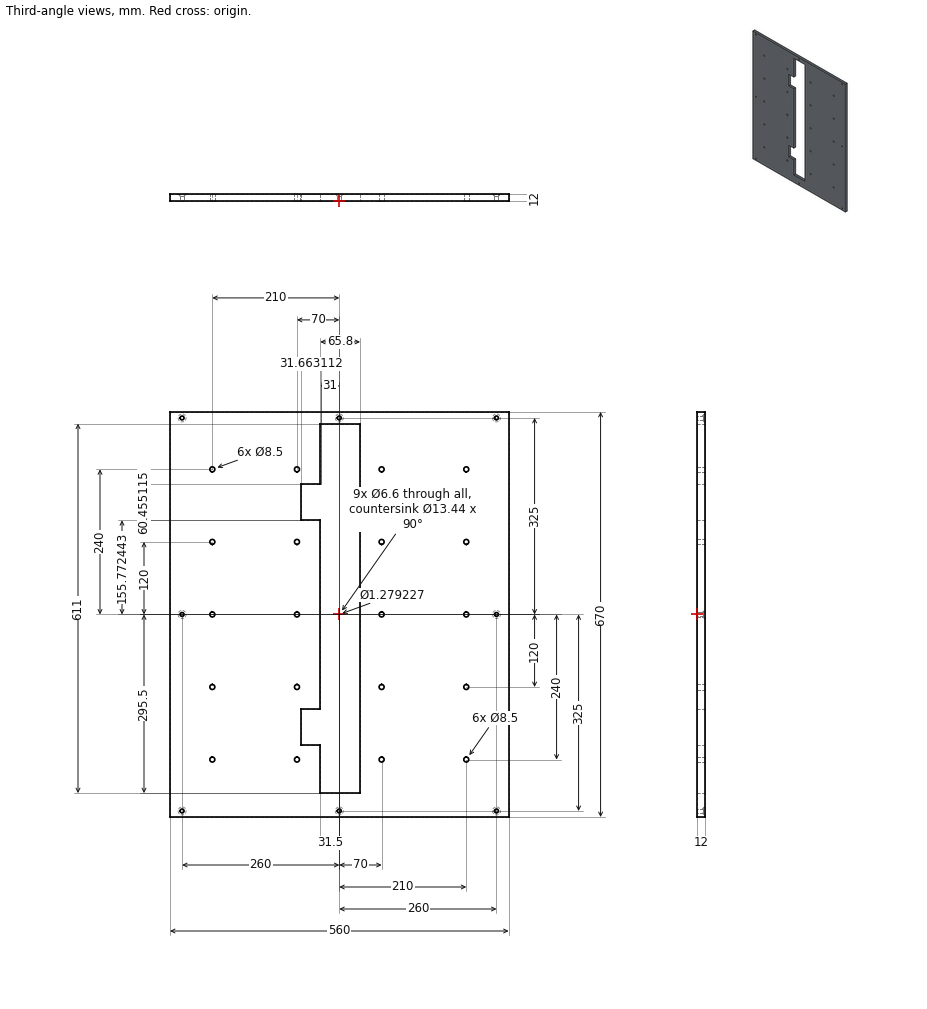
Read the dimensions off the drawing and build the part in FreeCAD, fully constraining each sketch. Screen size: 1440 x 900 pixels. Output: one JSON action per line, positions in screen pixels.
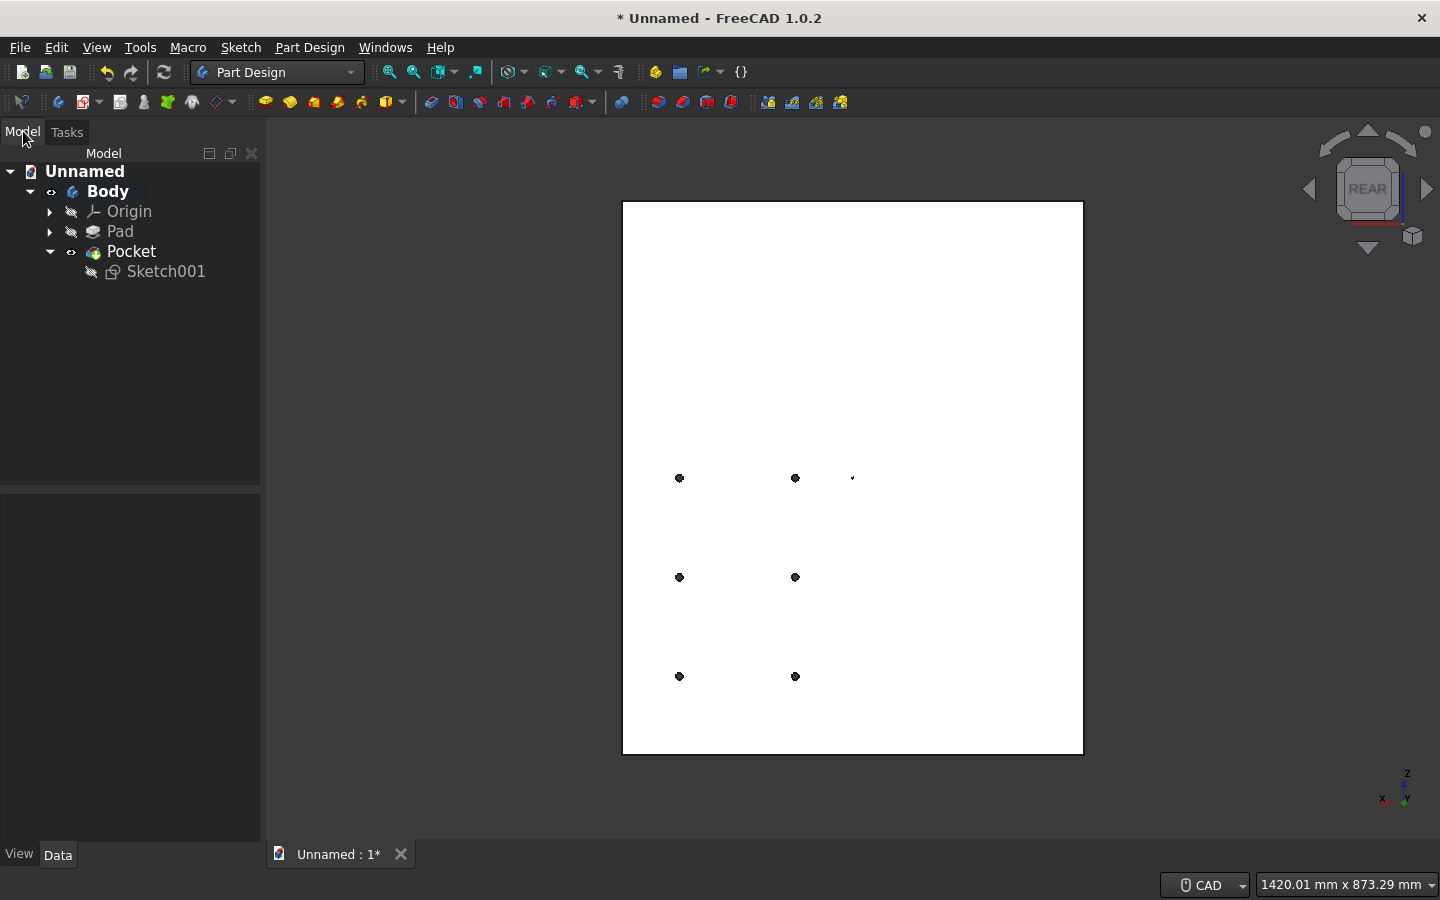
{"action": "left_click", "coordinate": [116, 252]}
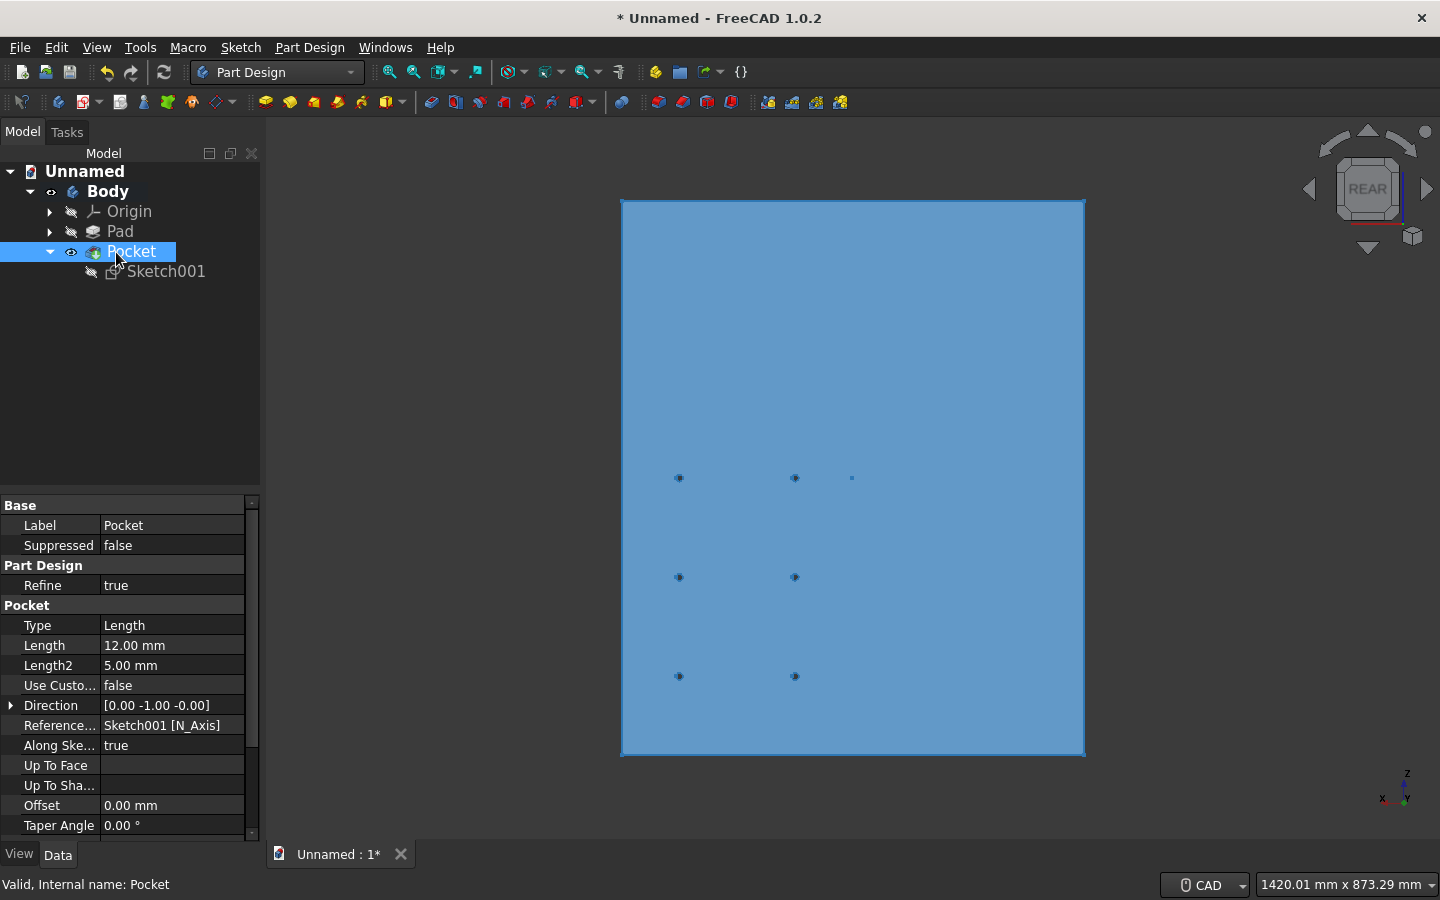
{"action": "left_click", "coordinate": [768, 102]}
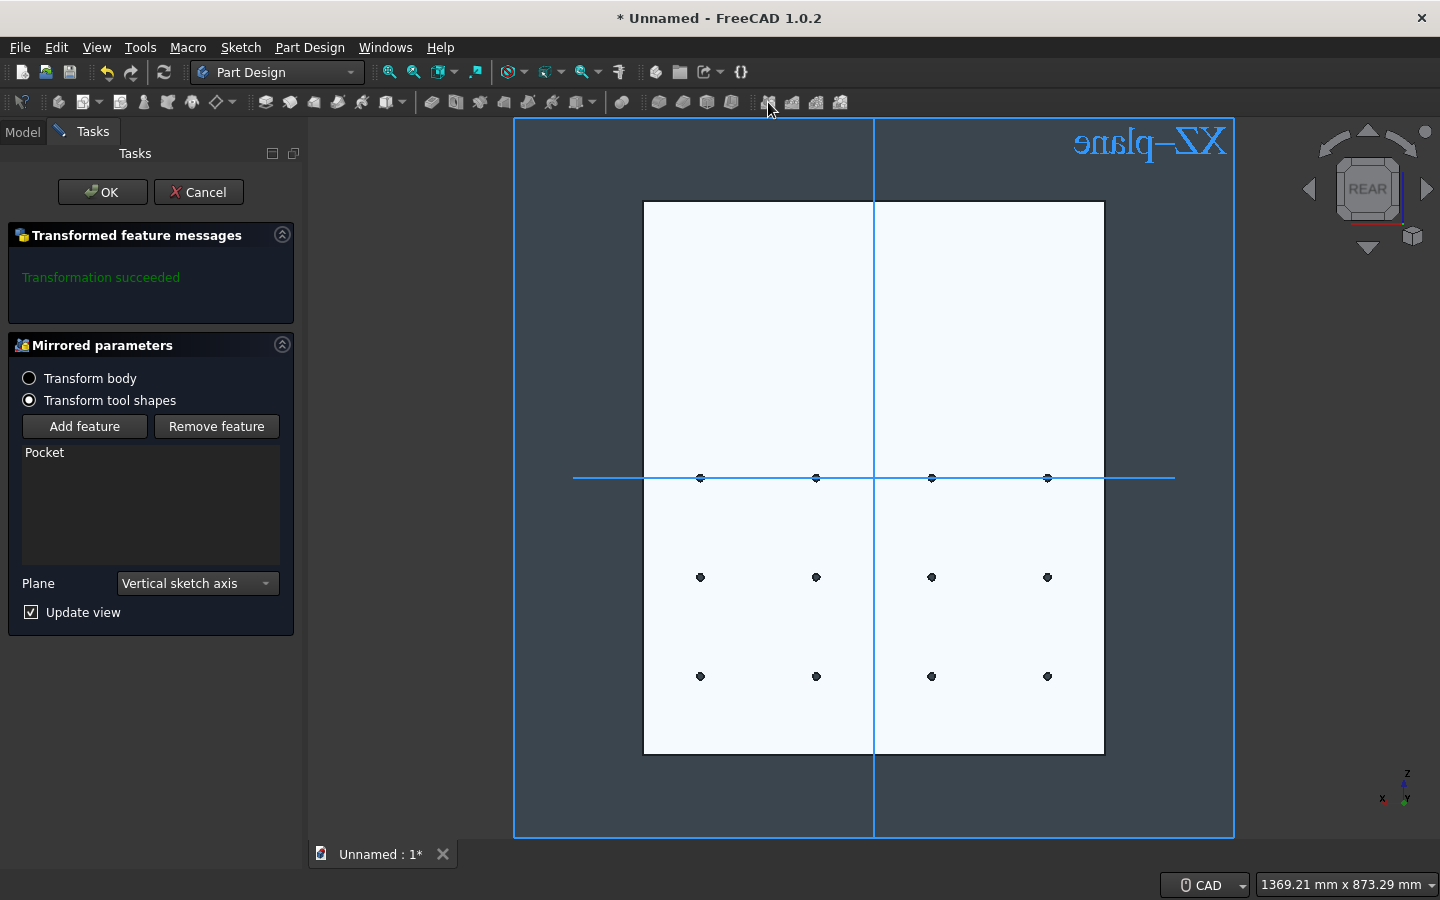
{"action": "left_click", "coordinate": [198, 584]}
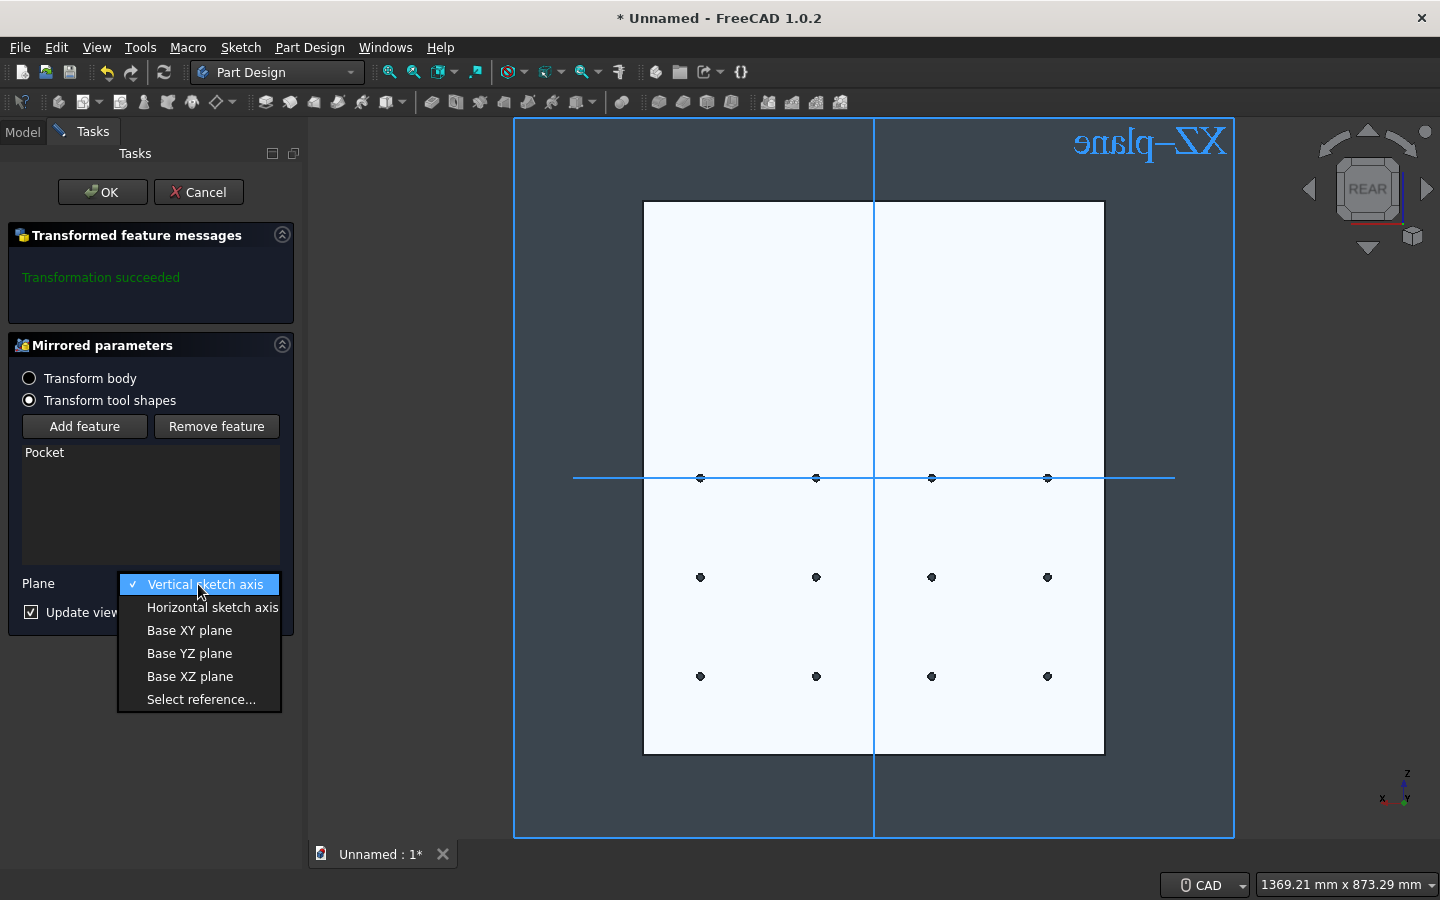
{"action": "left_click", "coordinate": [198, 654]}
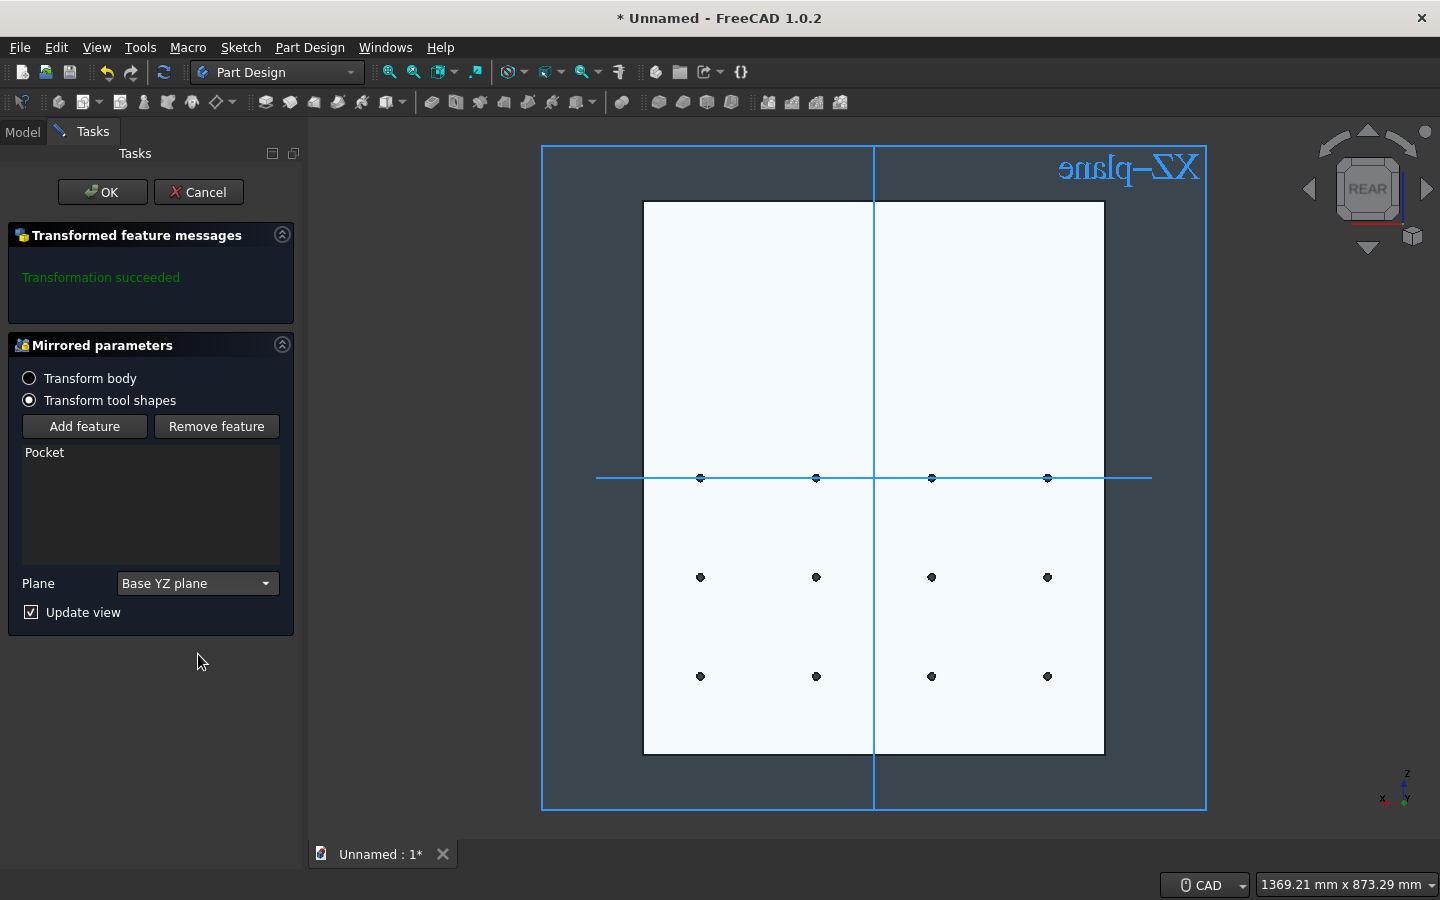
{"action": "left_click", "coordinate": [103, 192]}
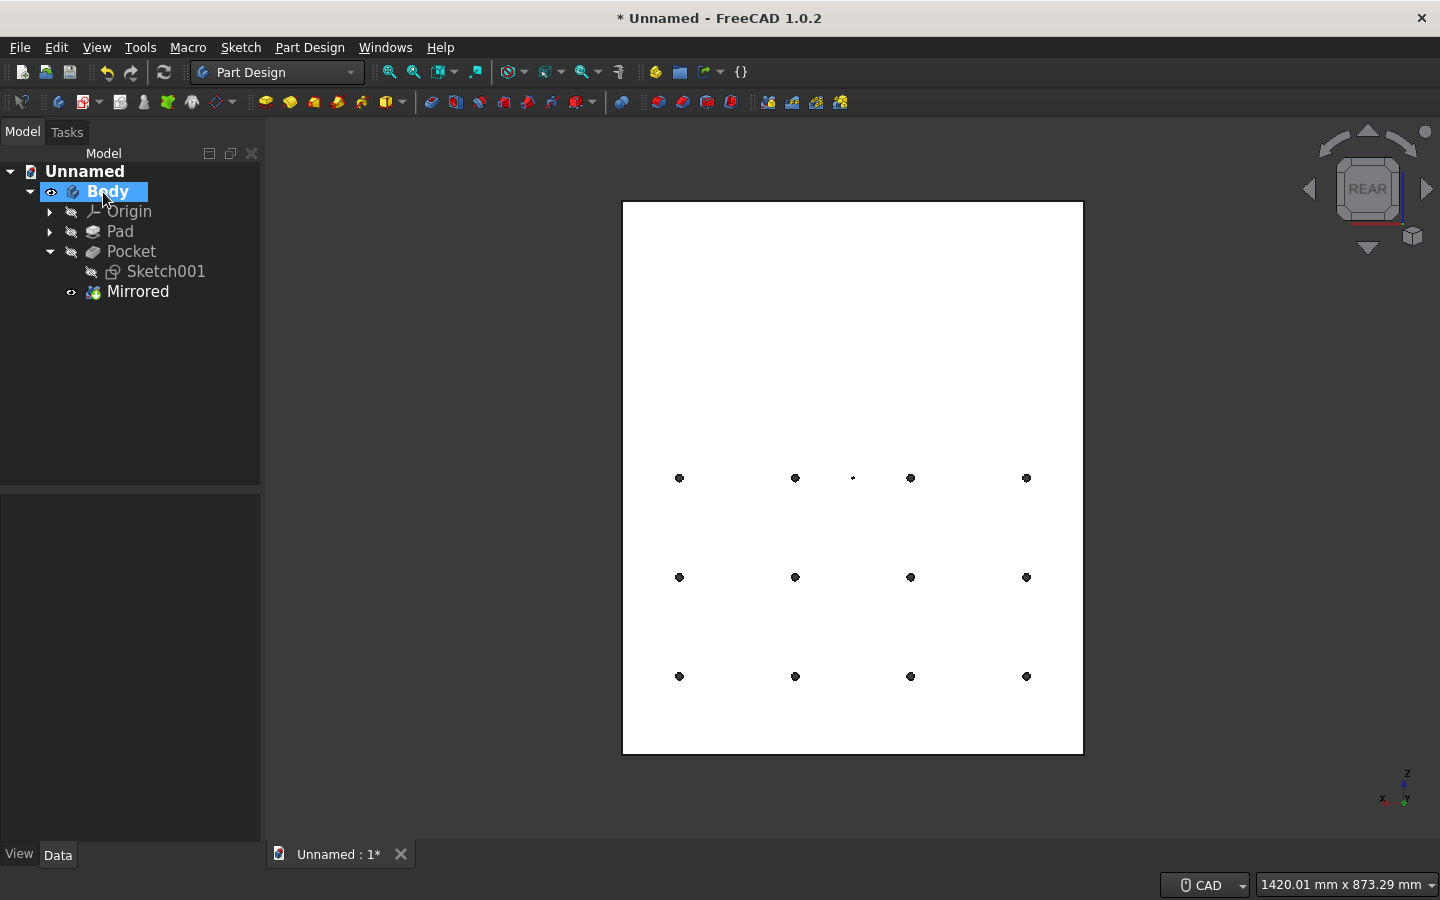
{"action": "left_click", "coordinate": [116, 252]}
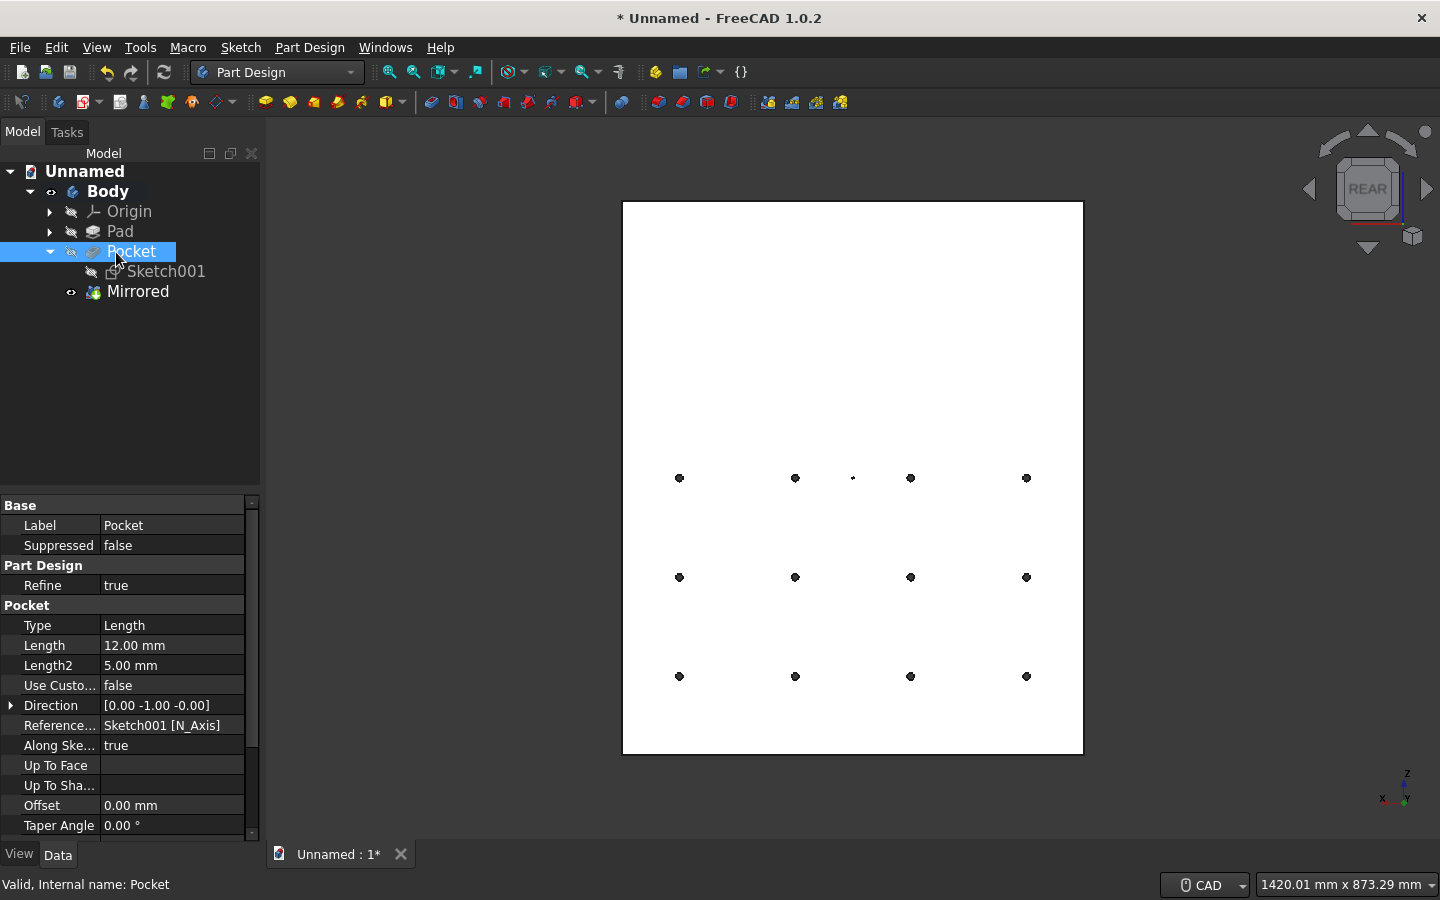
{"action": "left_click", "coordinate": [768, 102]}